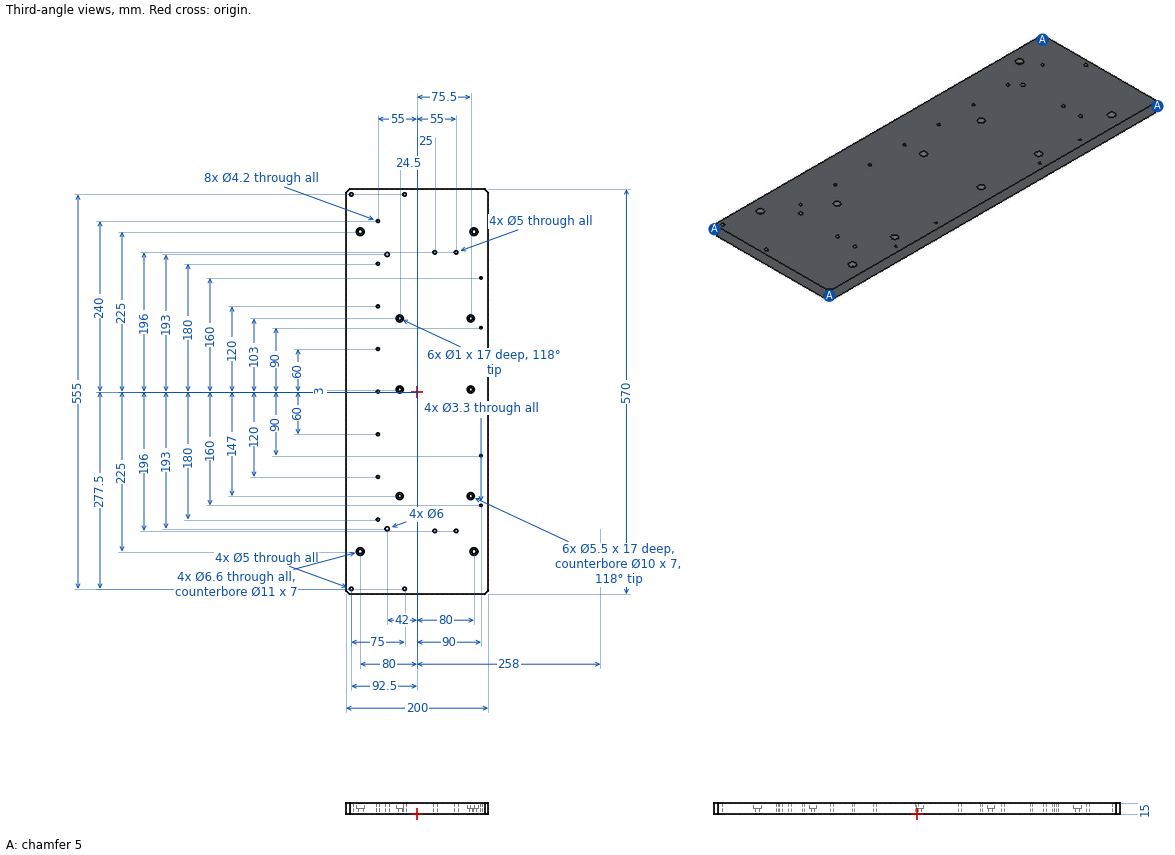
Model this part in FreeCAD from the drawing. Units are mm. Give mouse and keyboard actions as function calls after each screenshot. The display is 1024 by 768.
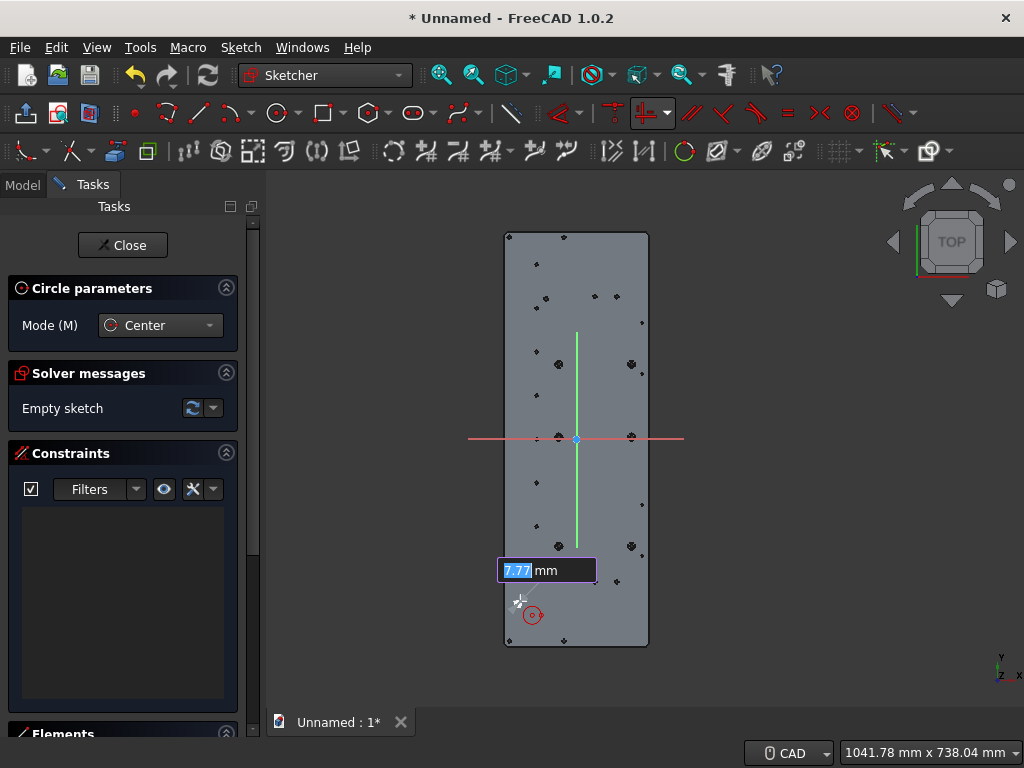
text(6.6)
key(Return)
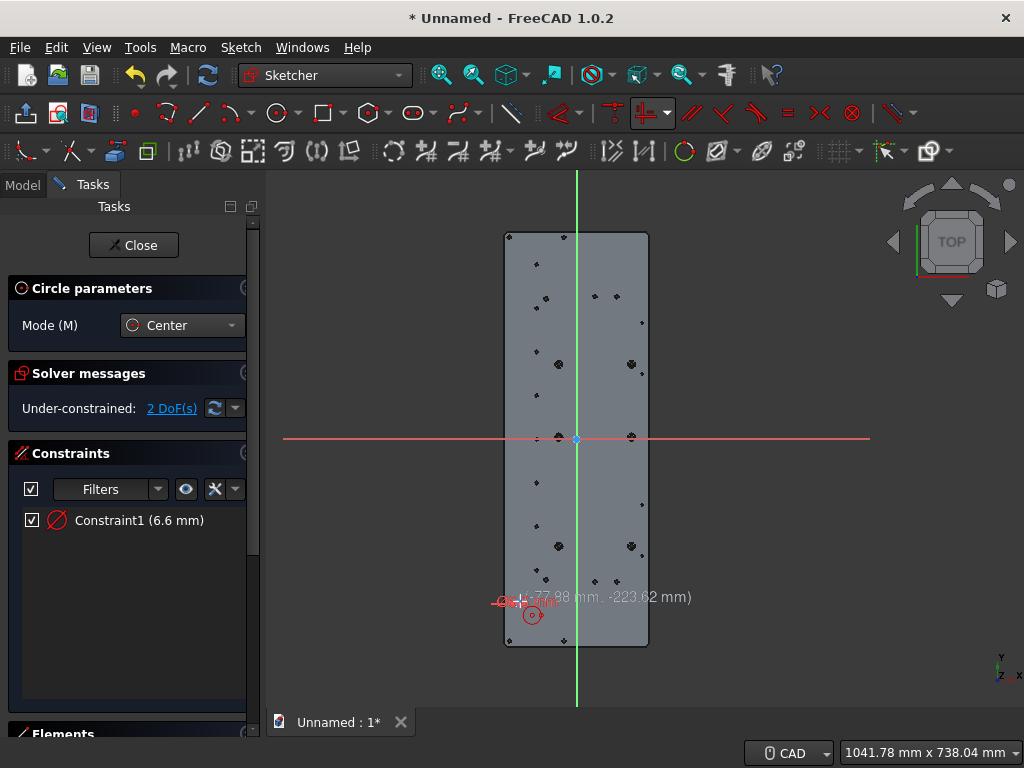
scroll(635, 603, up, 12)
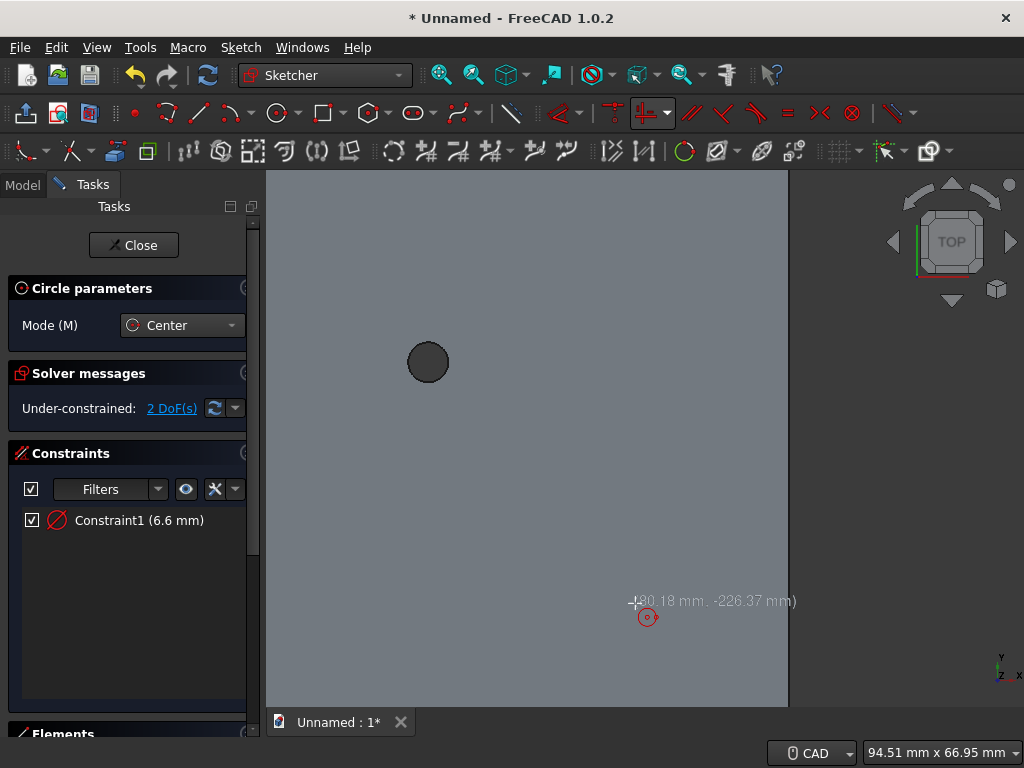
scroll(635, 603, down, 12)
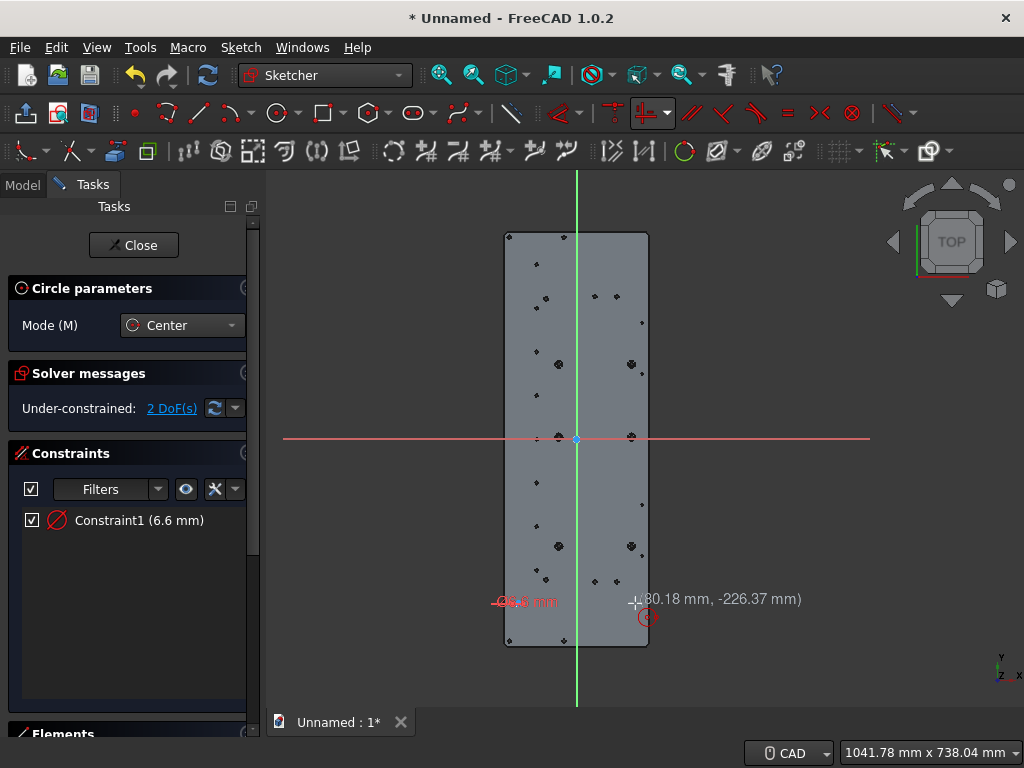
click(635, 603)
move(637, 601)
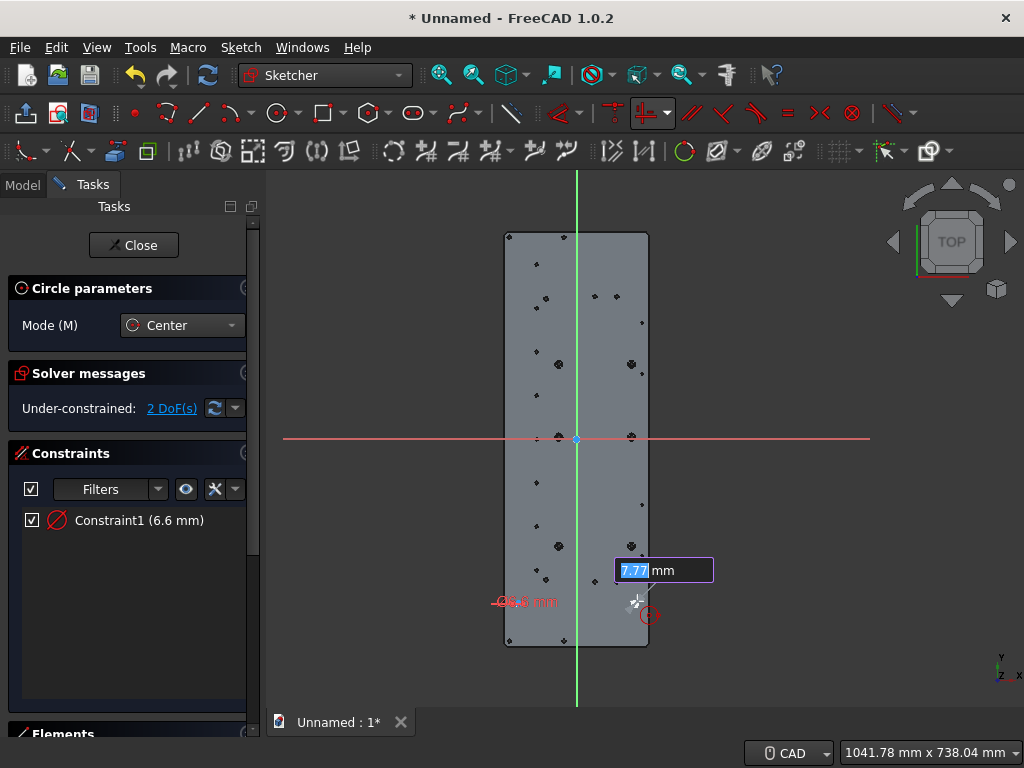
text(6.6)
key(Return)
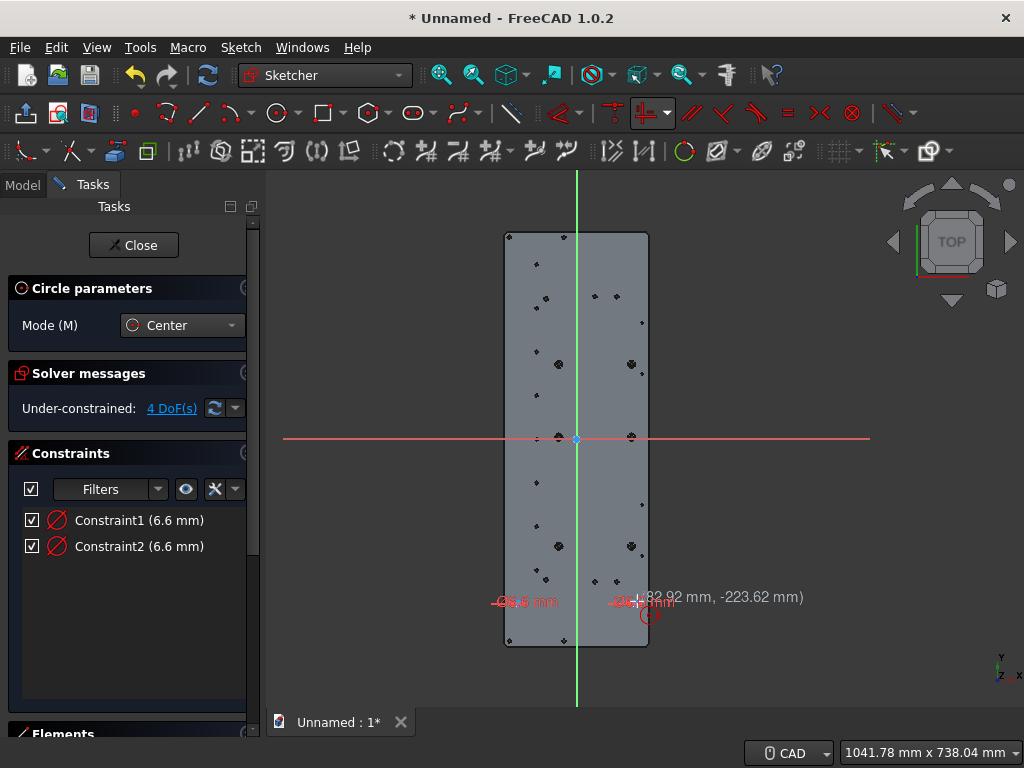
scroll(518, 276, up, 12)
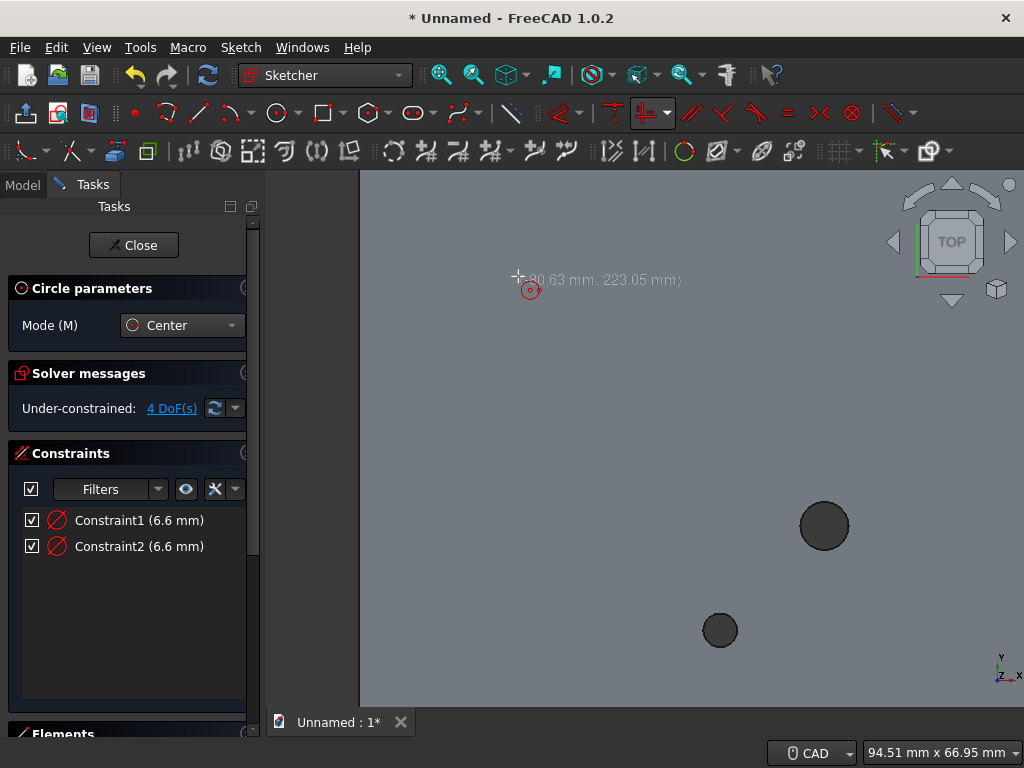
scroll(518, 275, down, 12)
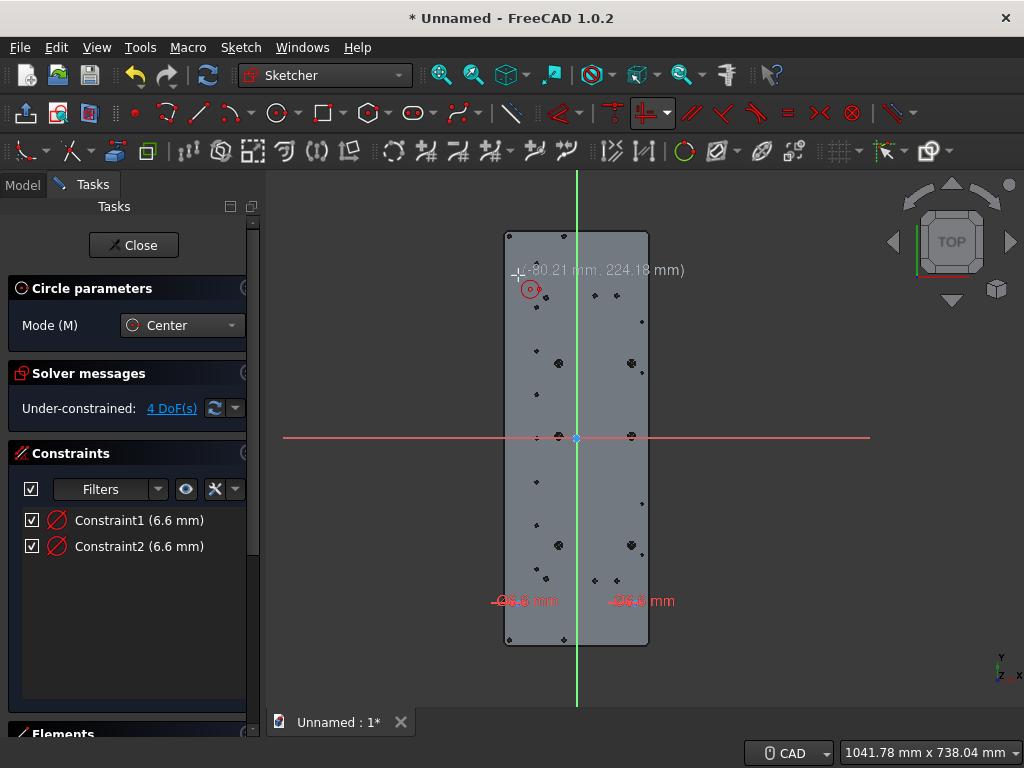
click(518, 275)
move(520, 273)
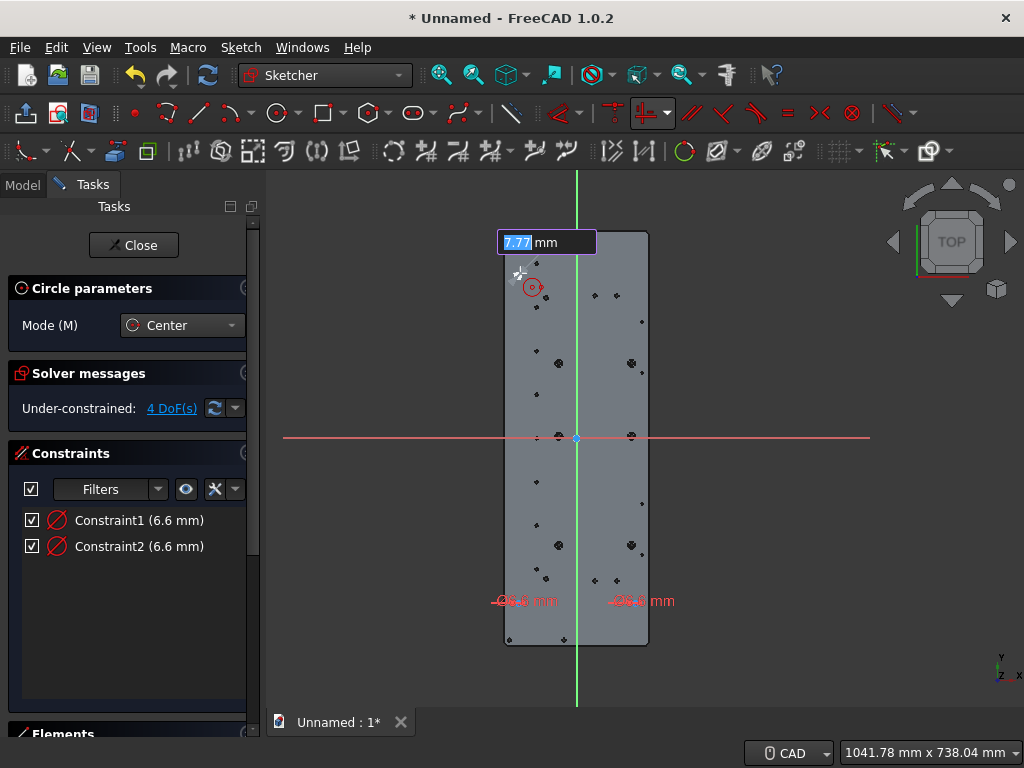
text(6.6)
key(Return)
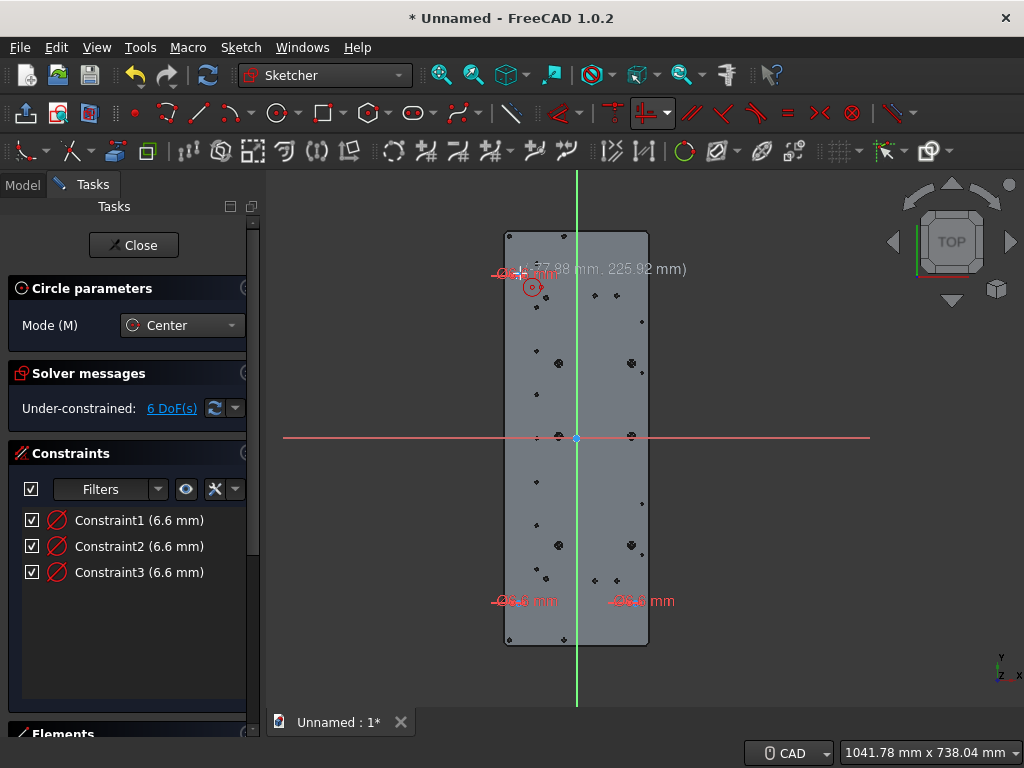
scroll(635, 275, up, 12)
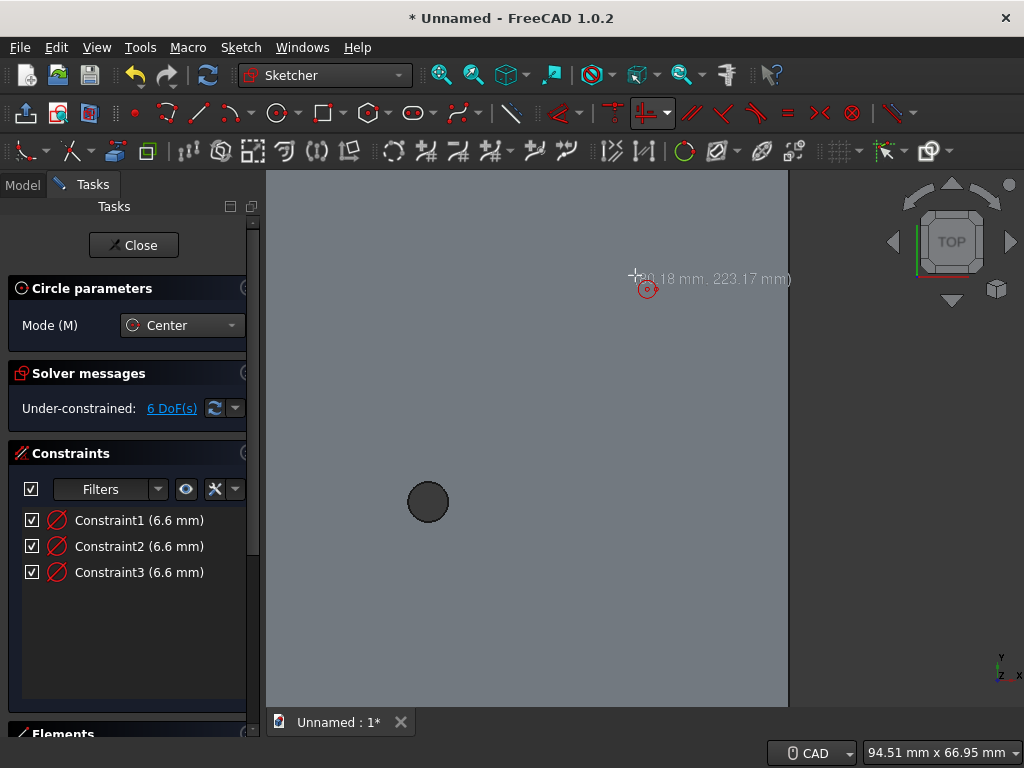
scroll(635, 275, down, 12)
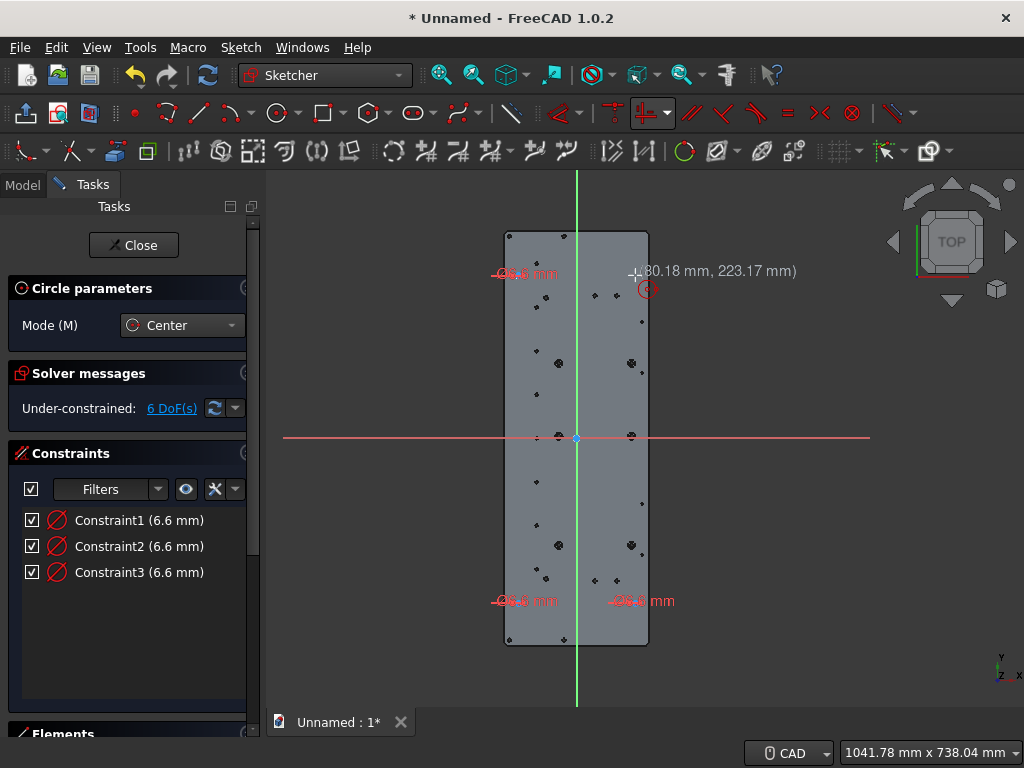
click(635, 275)
move(637, 273)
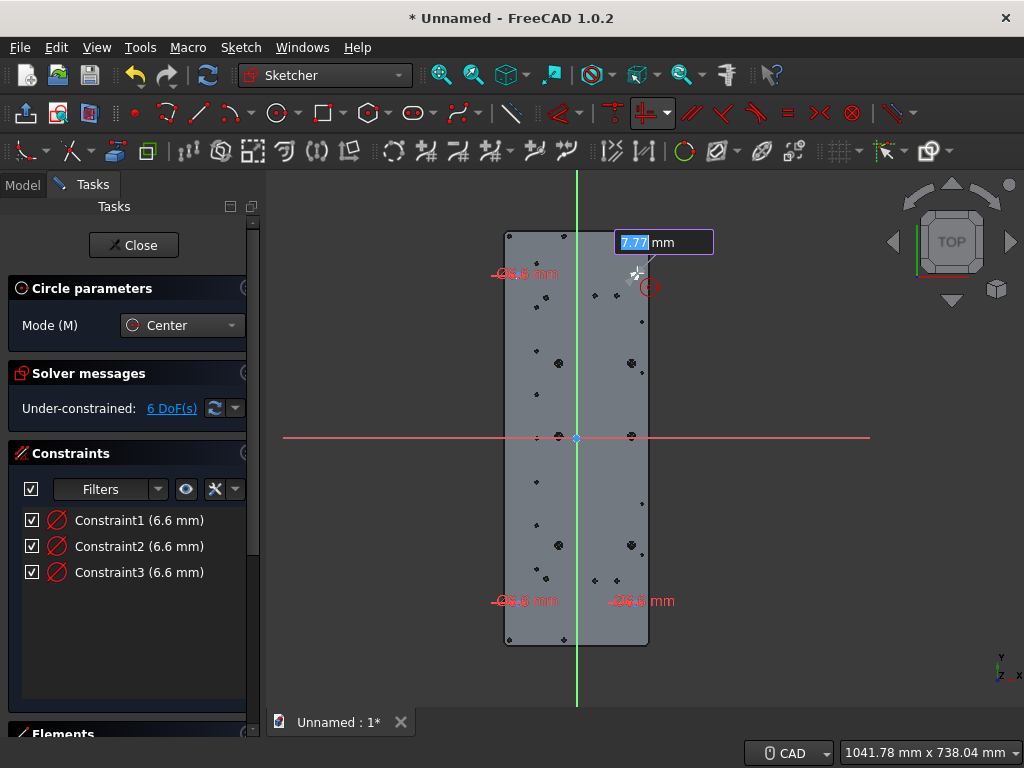
text(6.6)
key(Return)
key(Escape)